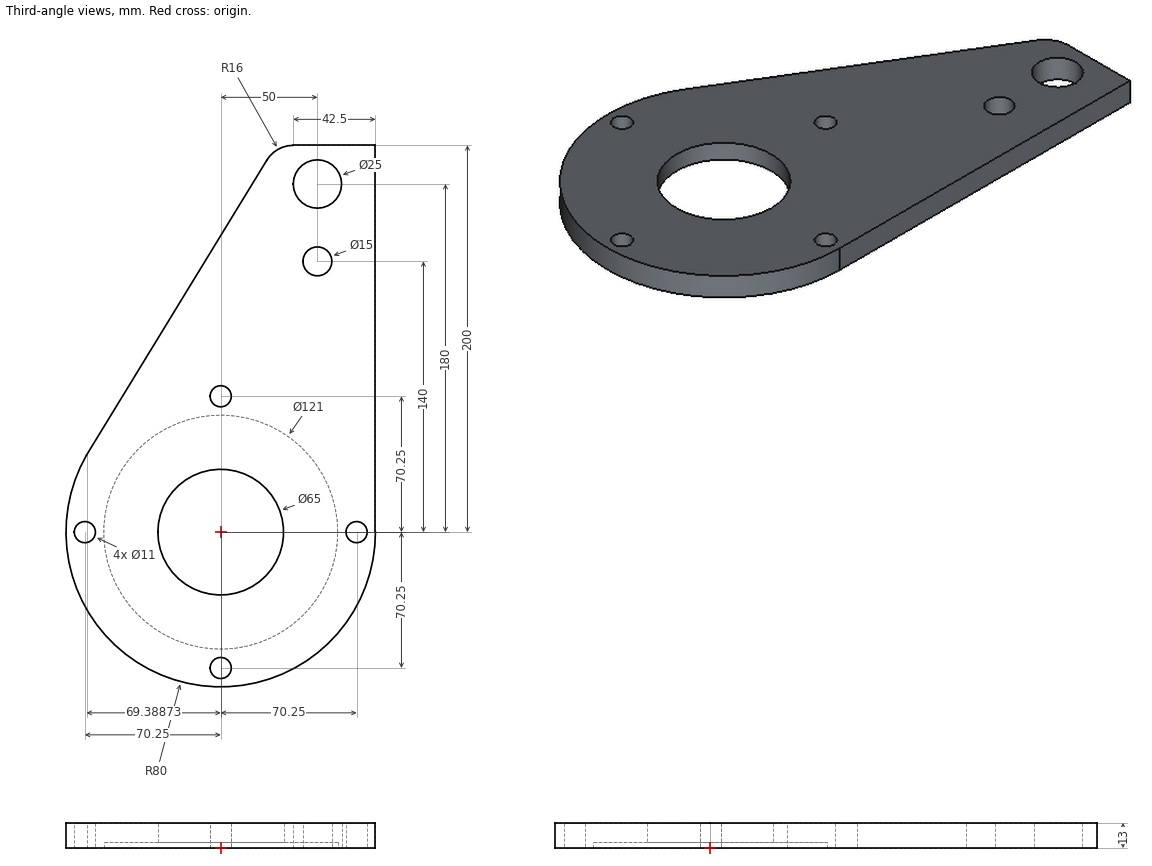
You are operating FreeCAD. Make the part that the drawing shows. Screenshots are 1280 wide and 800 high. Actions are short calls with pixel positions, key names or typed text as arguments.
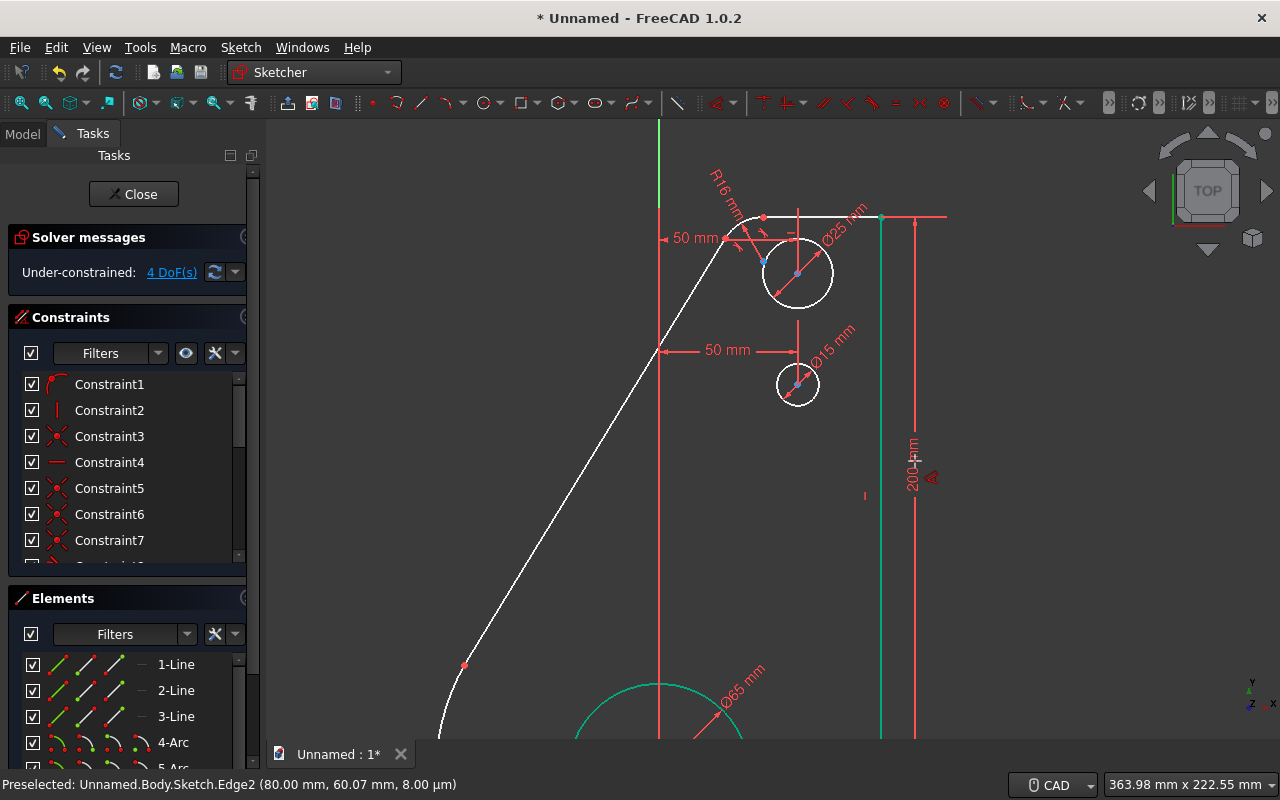
click(798, 385)
click(832, 548)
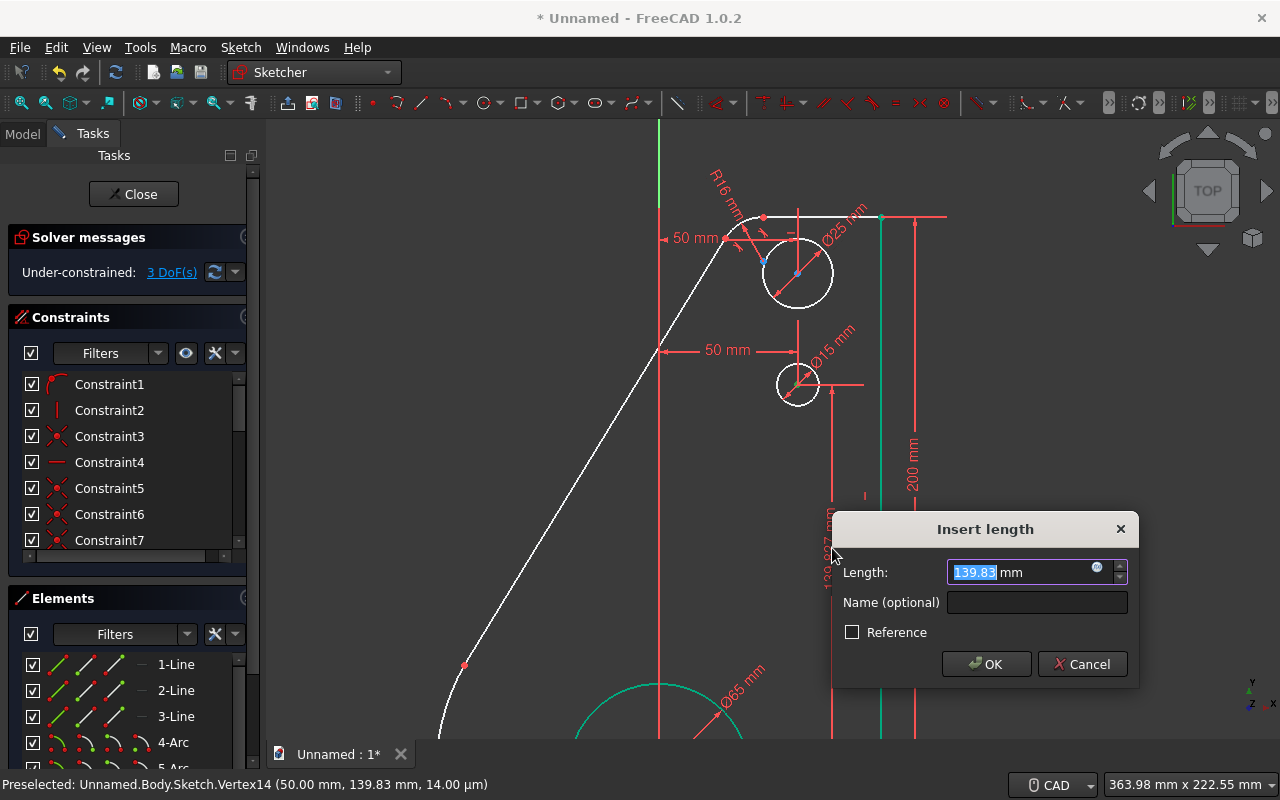
text(140)
key(Return)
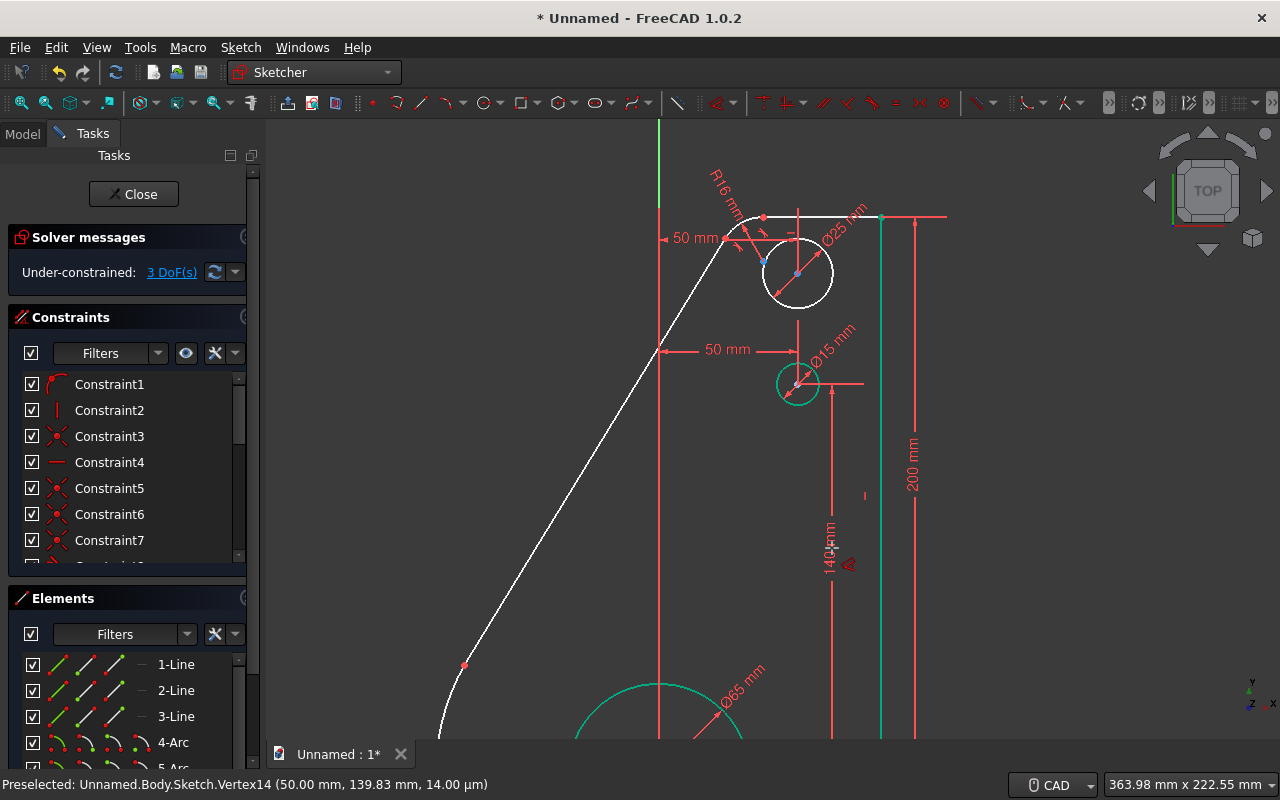
click(798, 273)
click(832, 492)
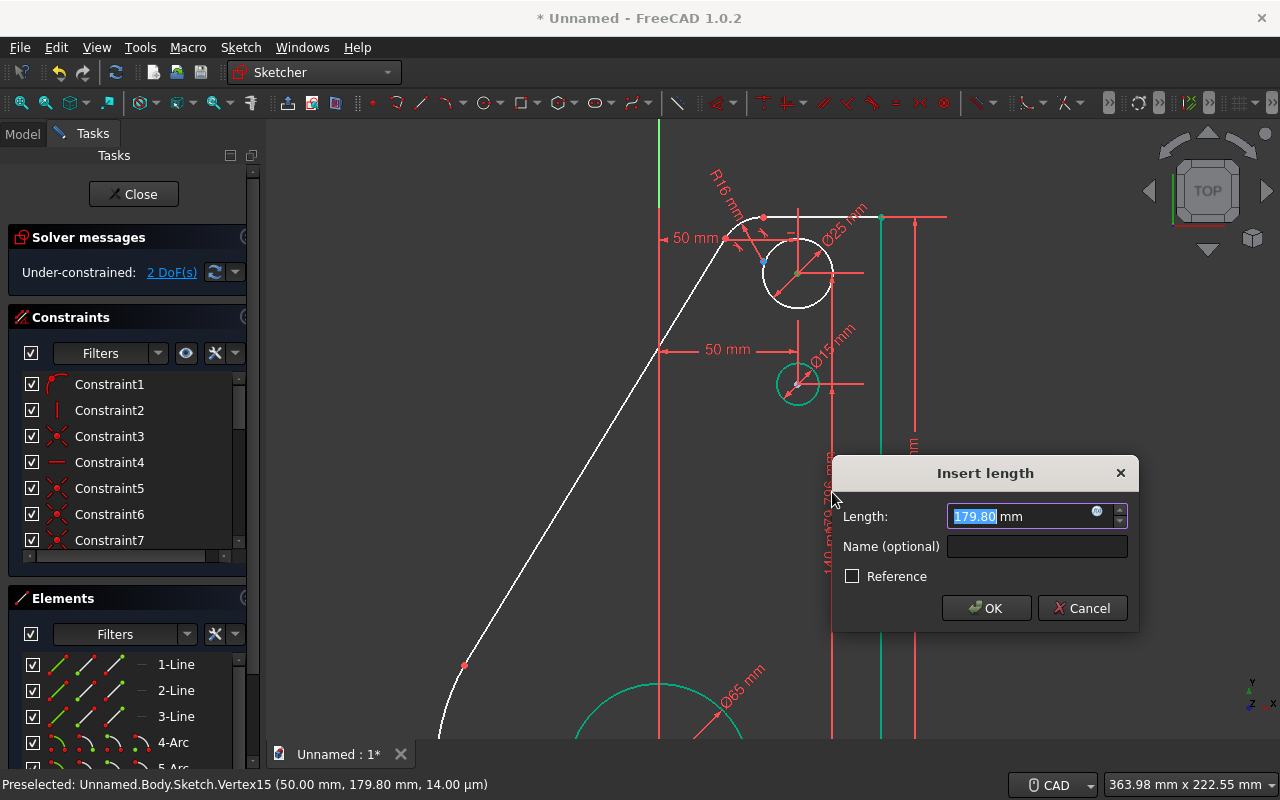
text(180)
key(Return)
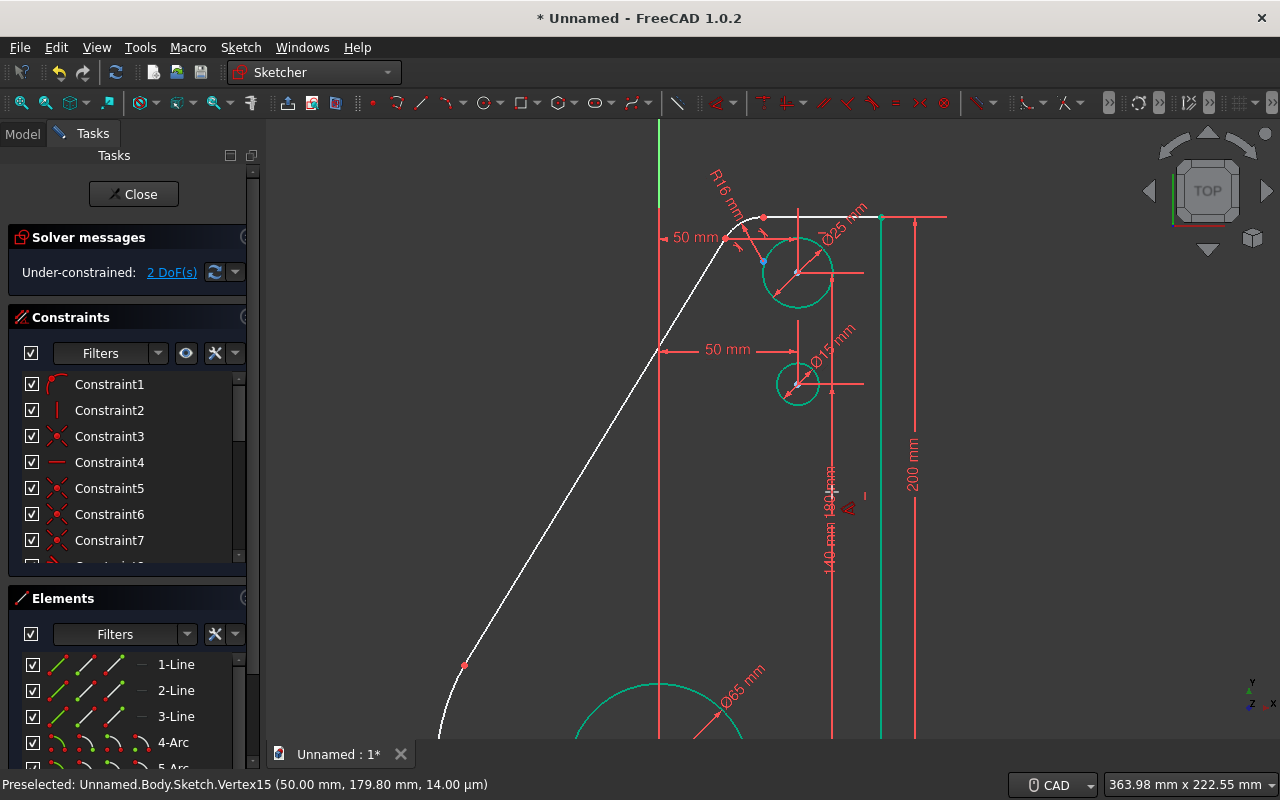
click(846, 217)
click(822, 183)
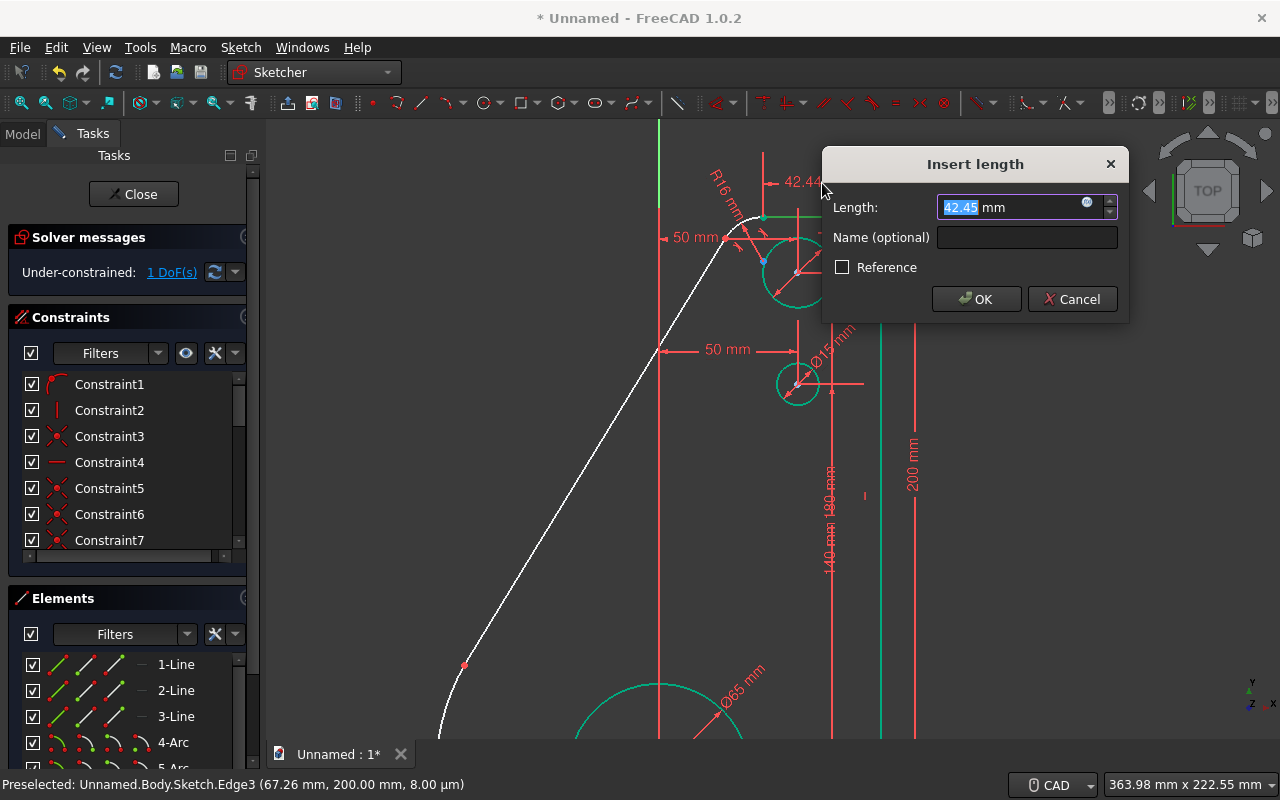
text(42.5)
key(Return)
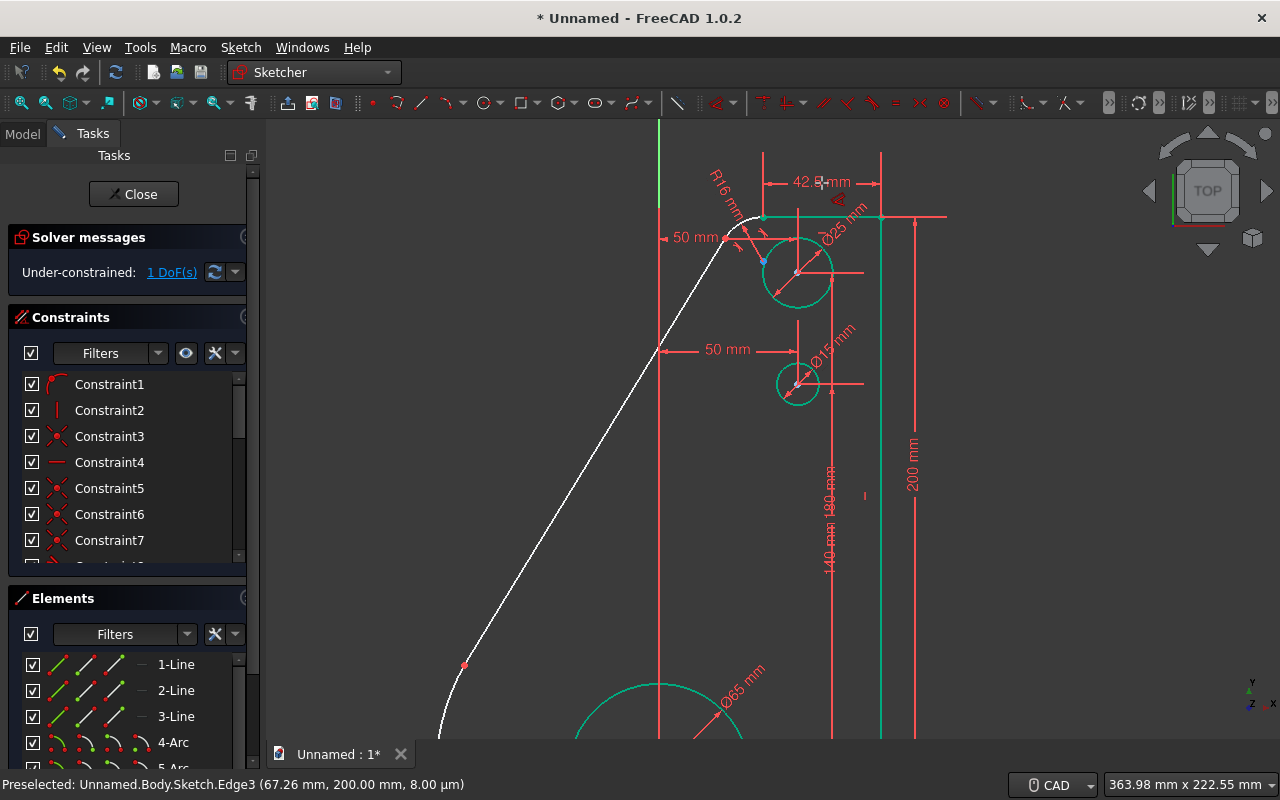
click(464, 665)
click(561, 631)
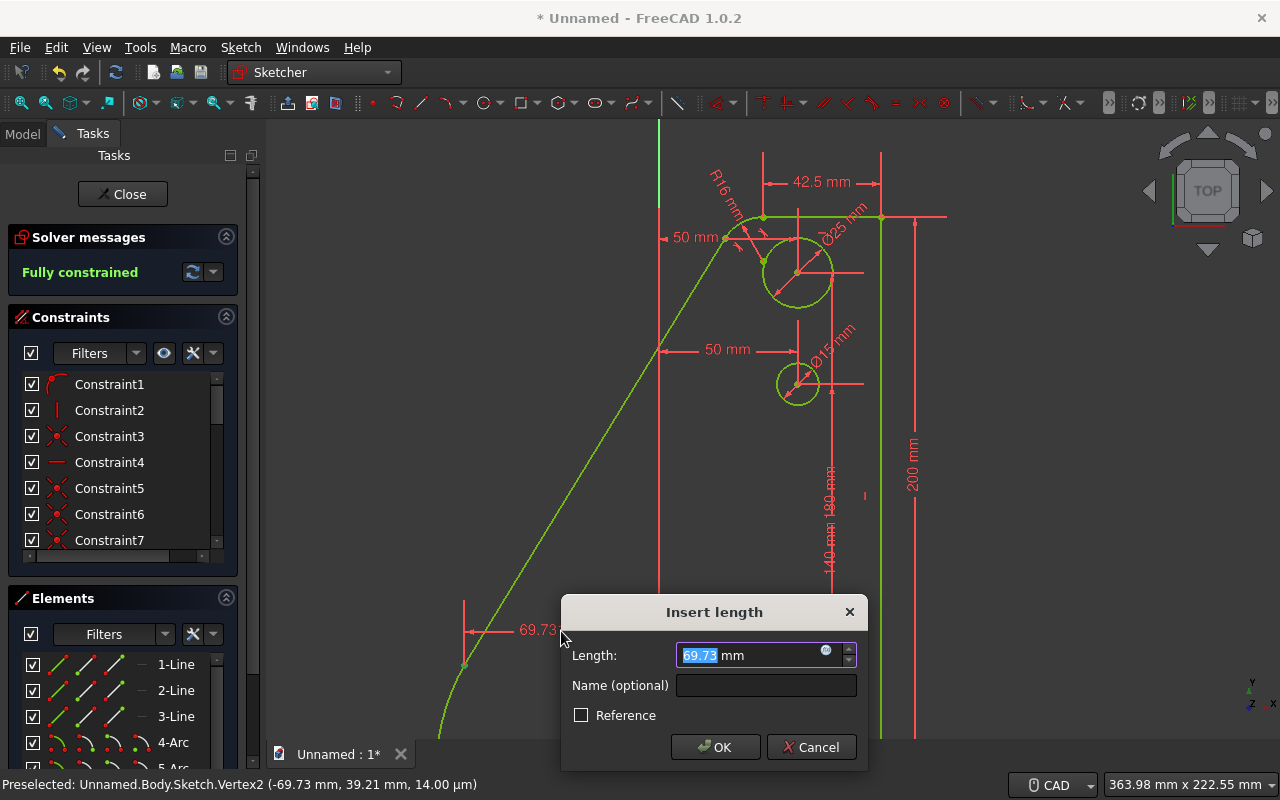
text(69.38873)
key(Return)
key(Escape)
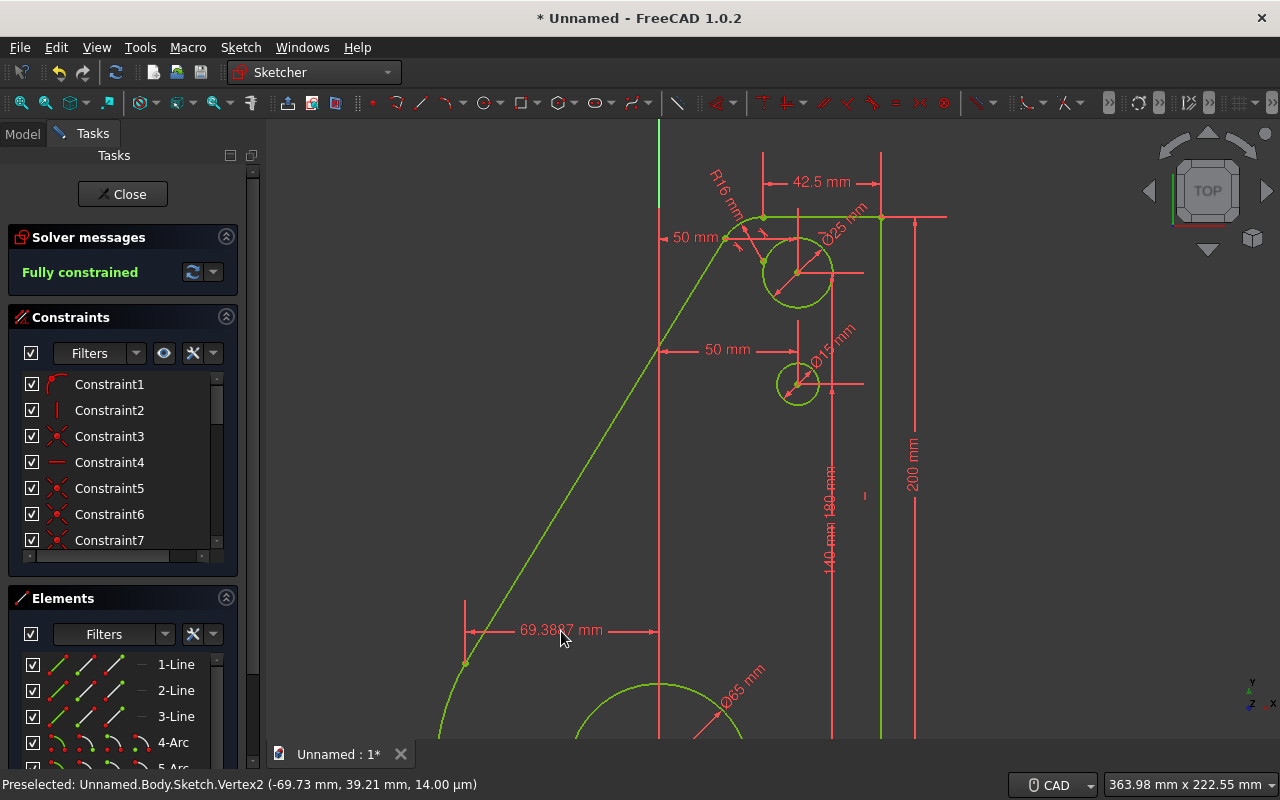
click(123, 194)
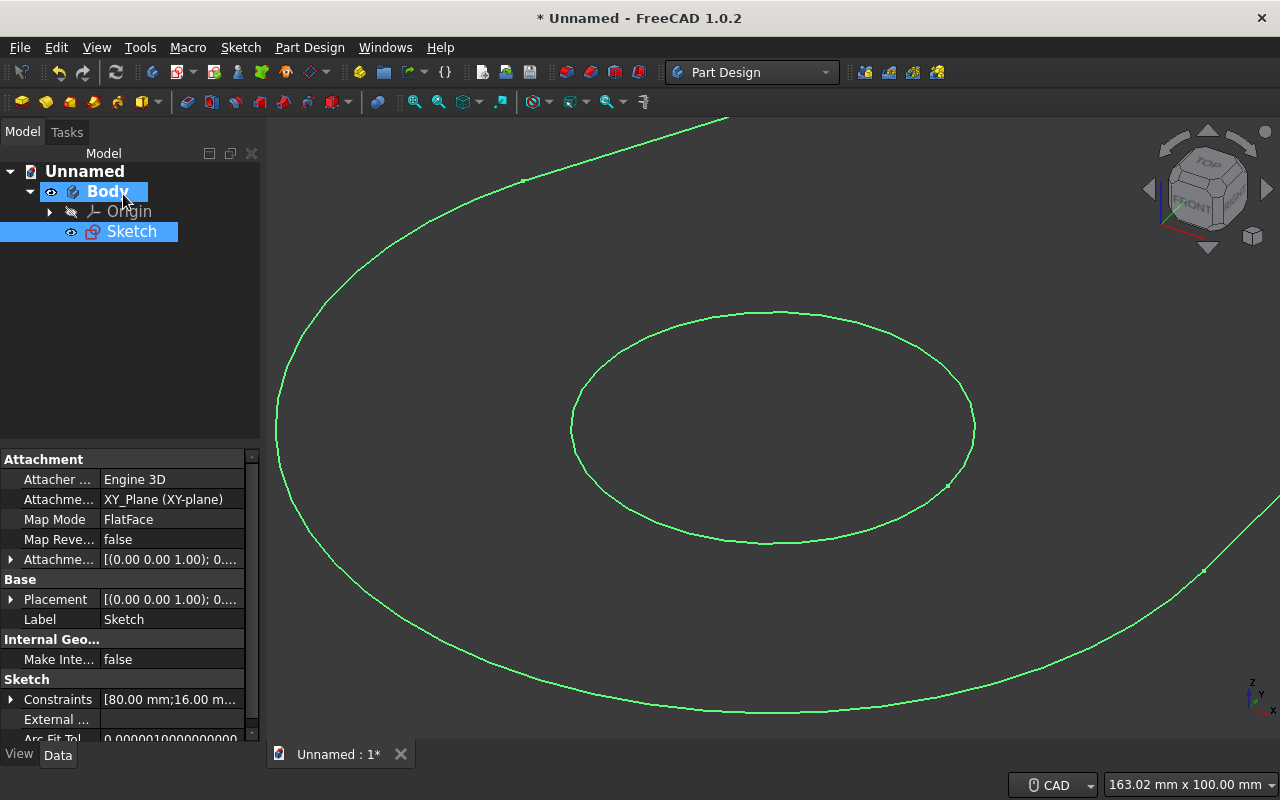
click(22, 102)